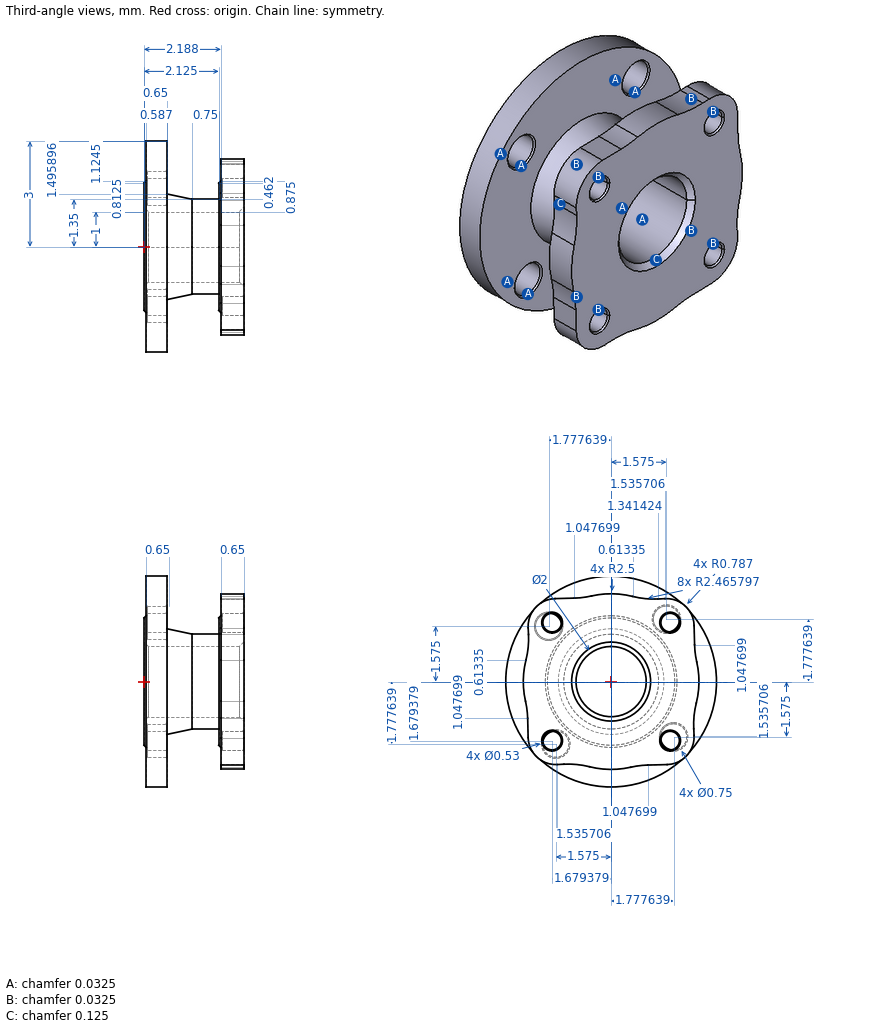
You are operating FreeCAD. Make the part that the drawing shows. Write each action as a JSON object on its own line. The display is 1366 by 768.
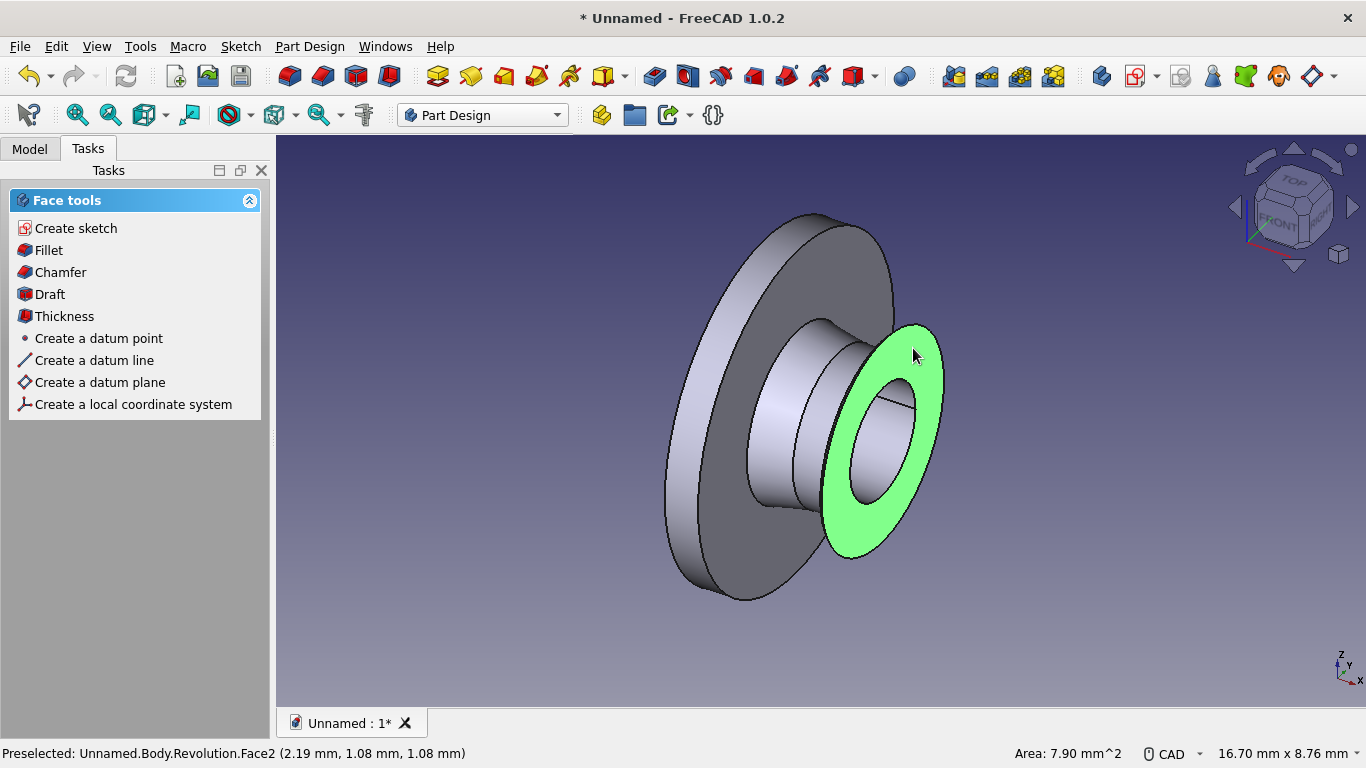
{"action": "left_click", "coordinate": [1134, 76]}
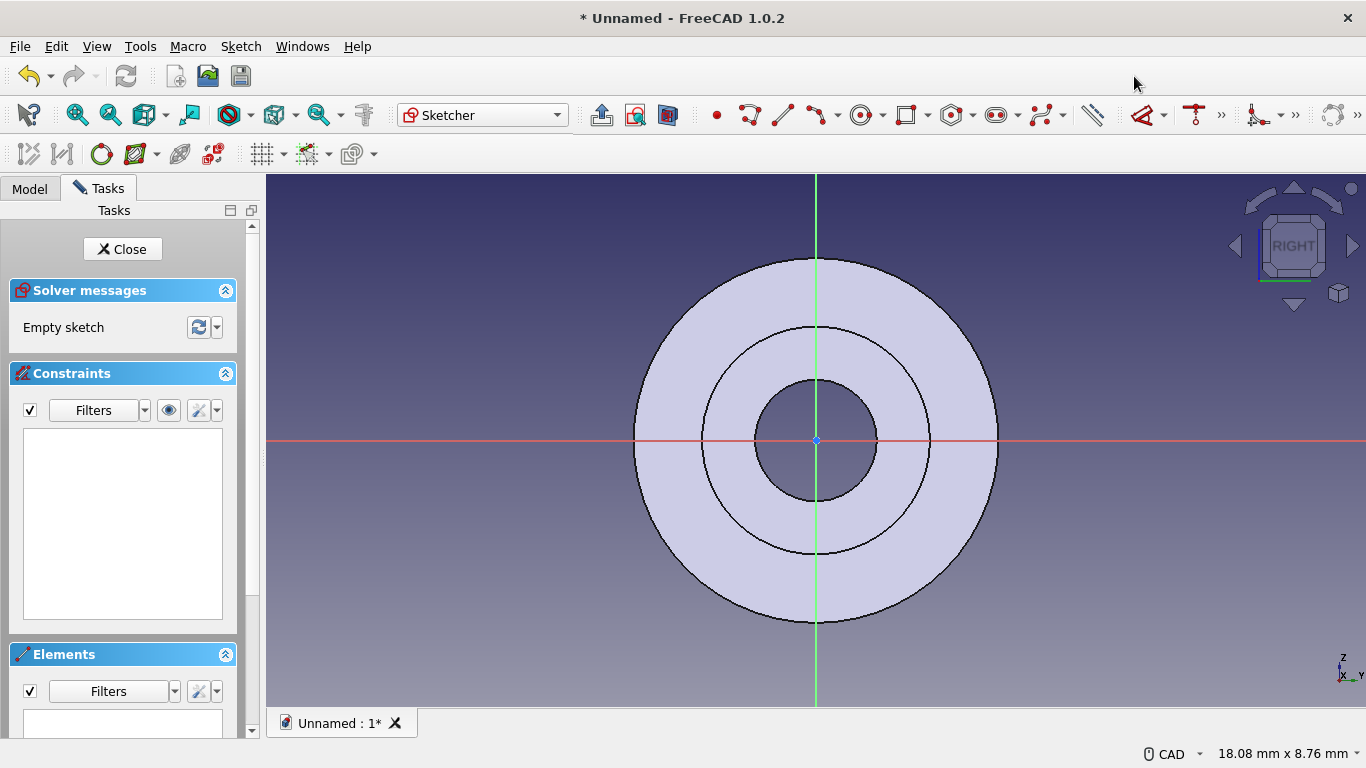
{"action": "left_click", "coordinate": [783, 116]}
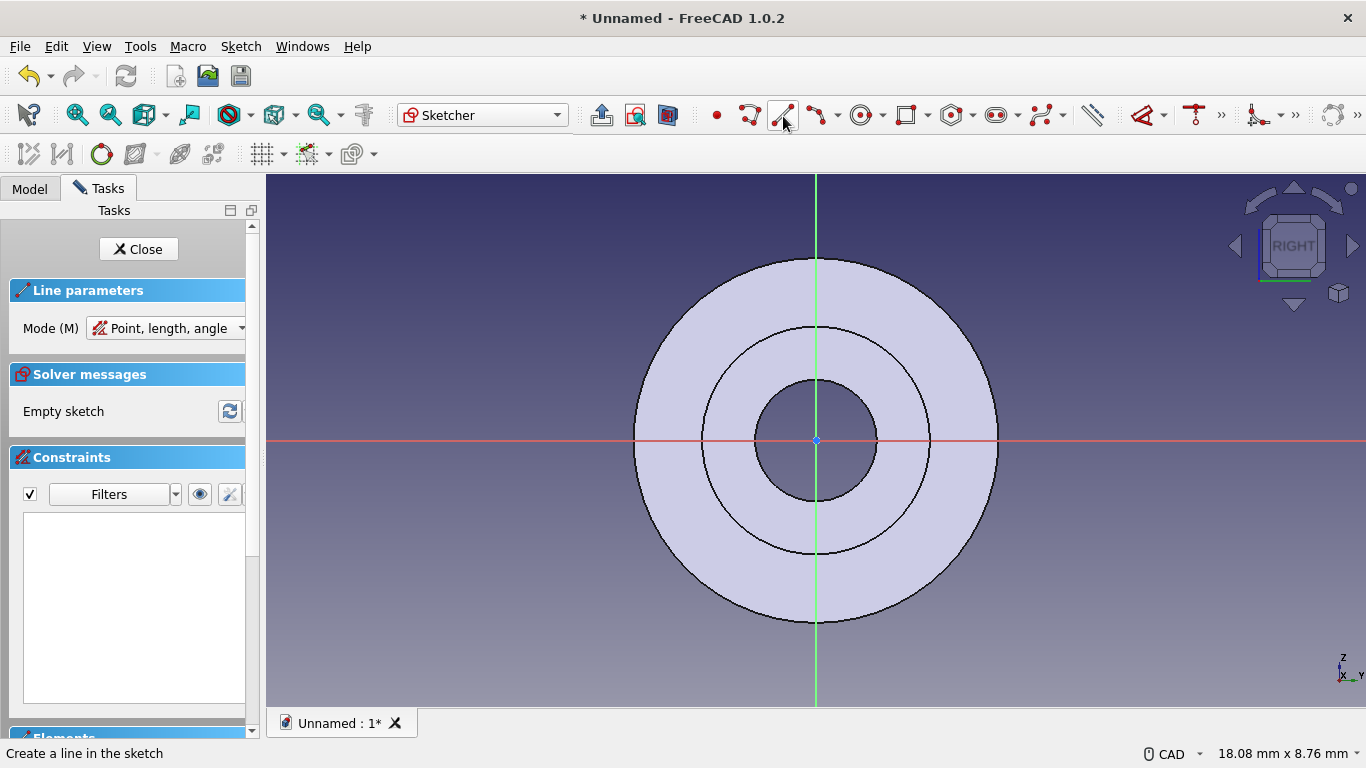
{"action": "left_click", "coordinate": [960, 377]}
{"action": "left_click", "coordinate": [957, 344]}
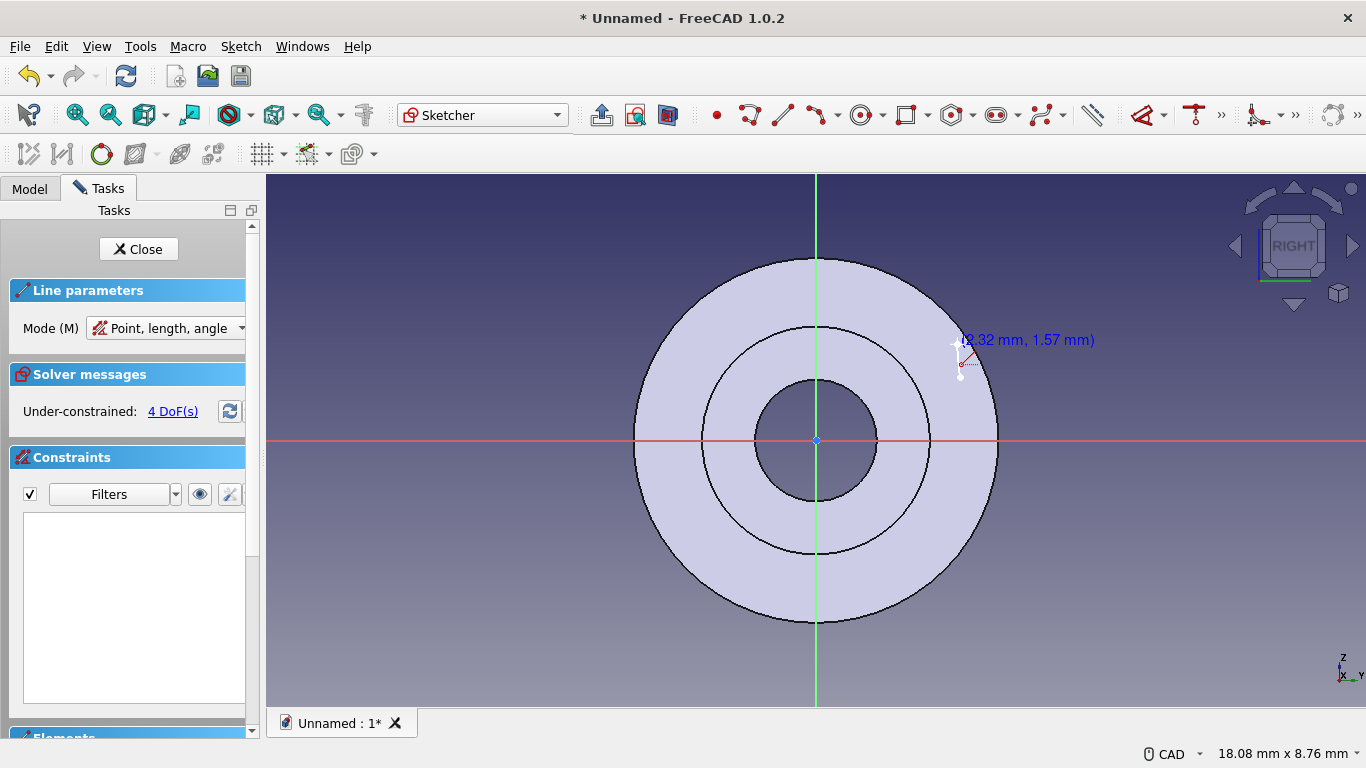
{"action": "left_click", "coordinate": [909, 297]}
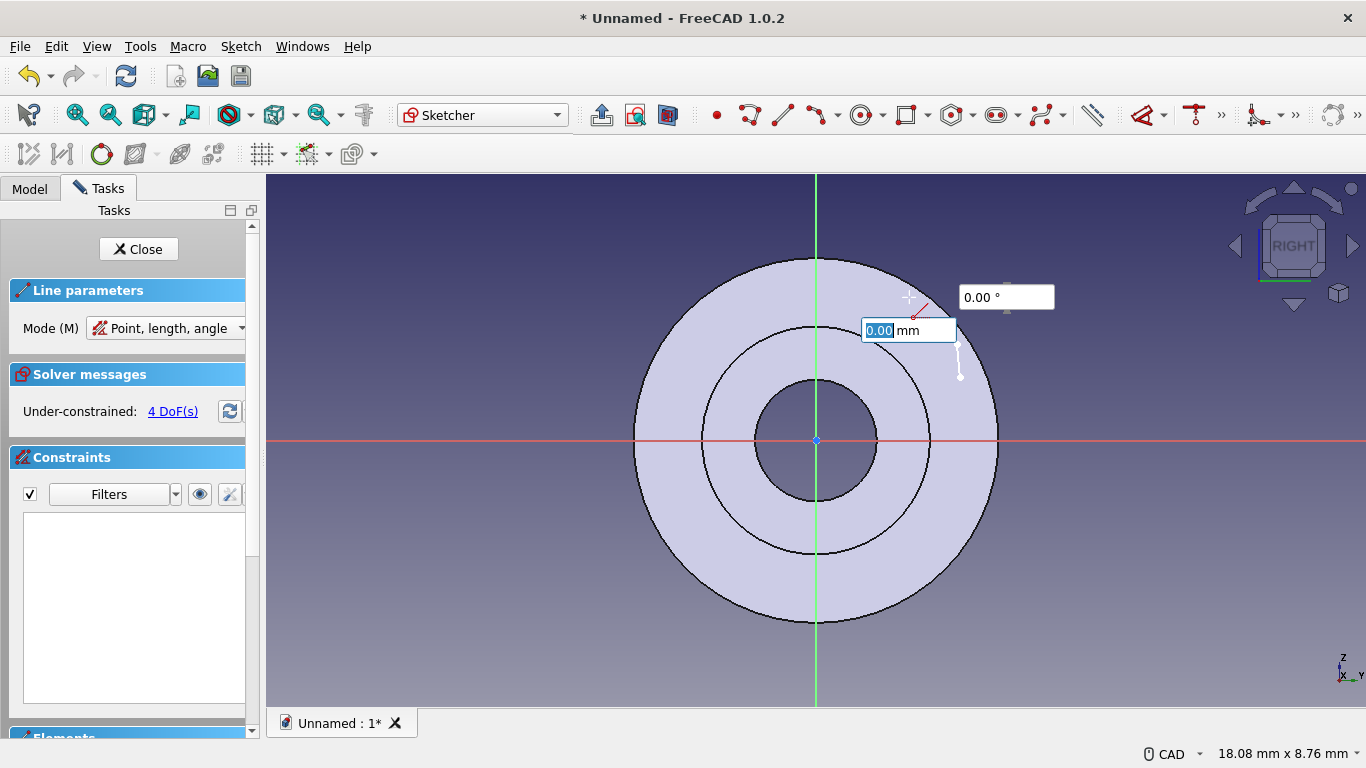
{"action": "scroll", "coordinate": [898, 297], "scroll_direction": "up", "scroll_amount": 2}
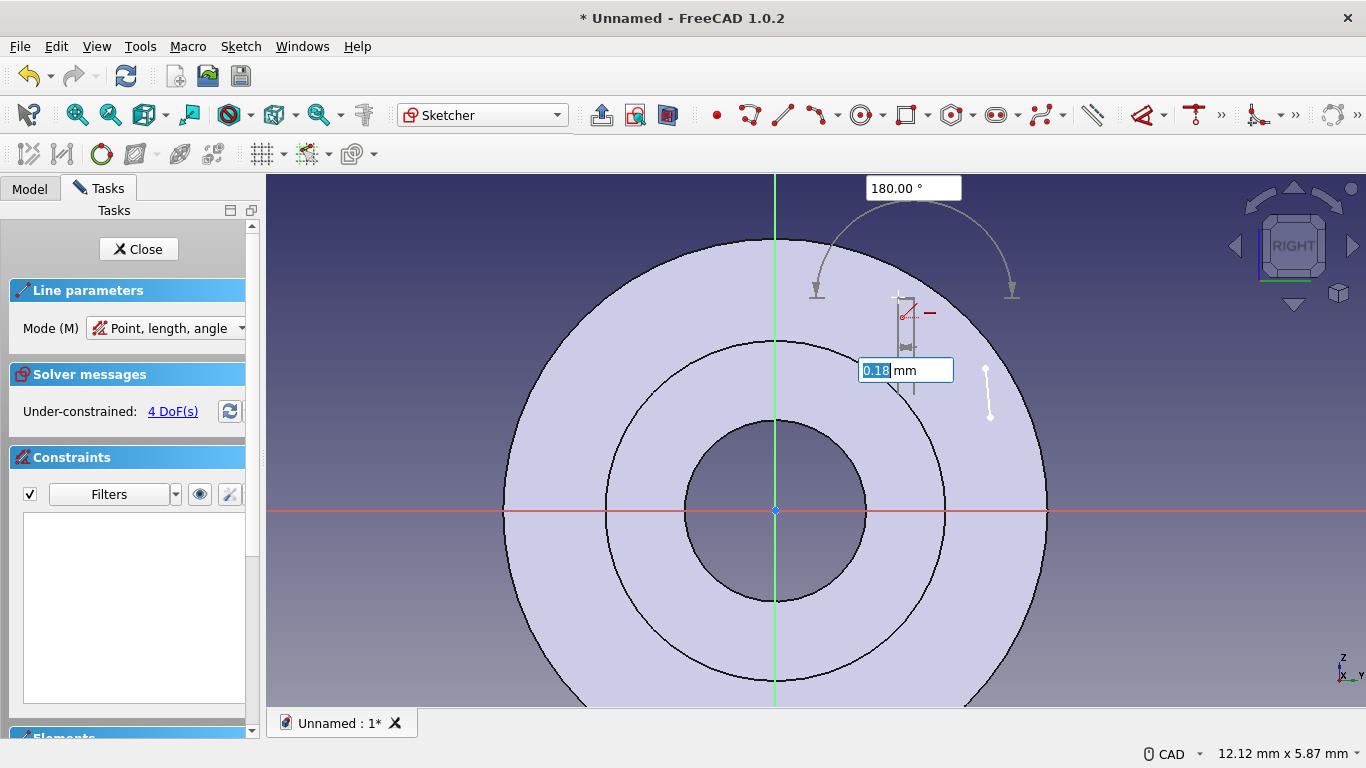
{"action": "left_click", "coordinate": [897, 299]}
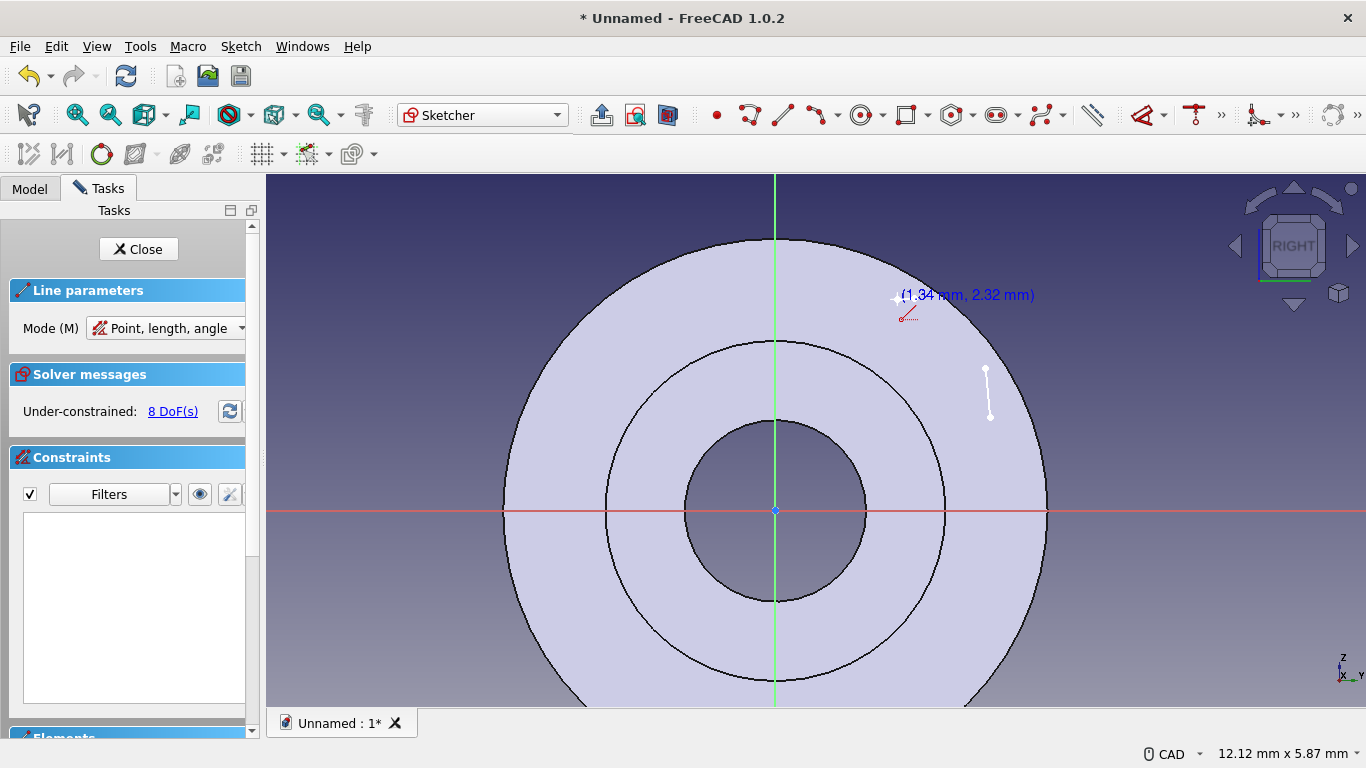
{"action": "left_click", "coordinate": [680, 295]}
{"action": "left_click", "coordinate": [631, 299]}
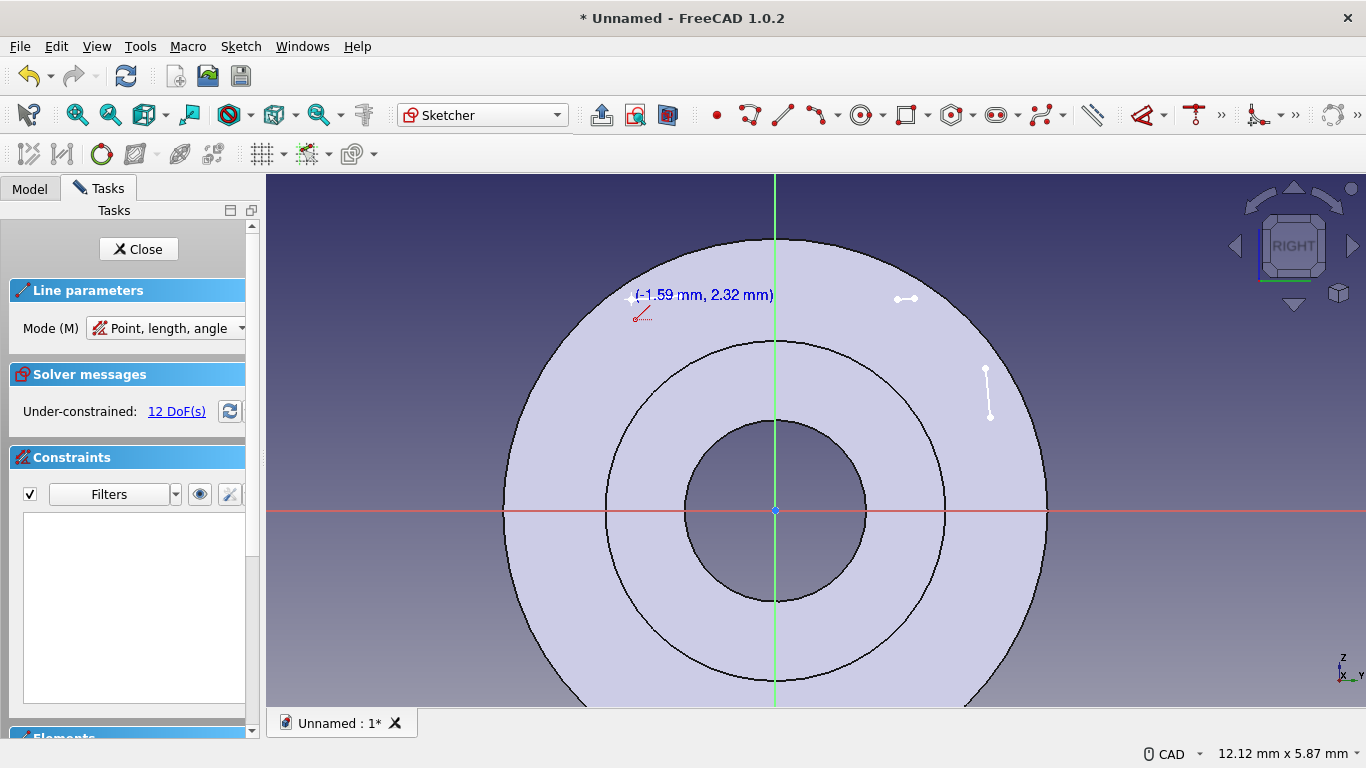
{"action": "left_click", "coordinate": [561, 372]}
{"action": "left_click", "coordinate": [563, 389]}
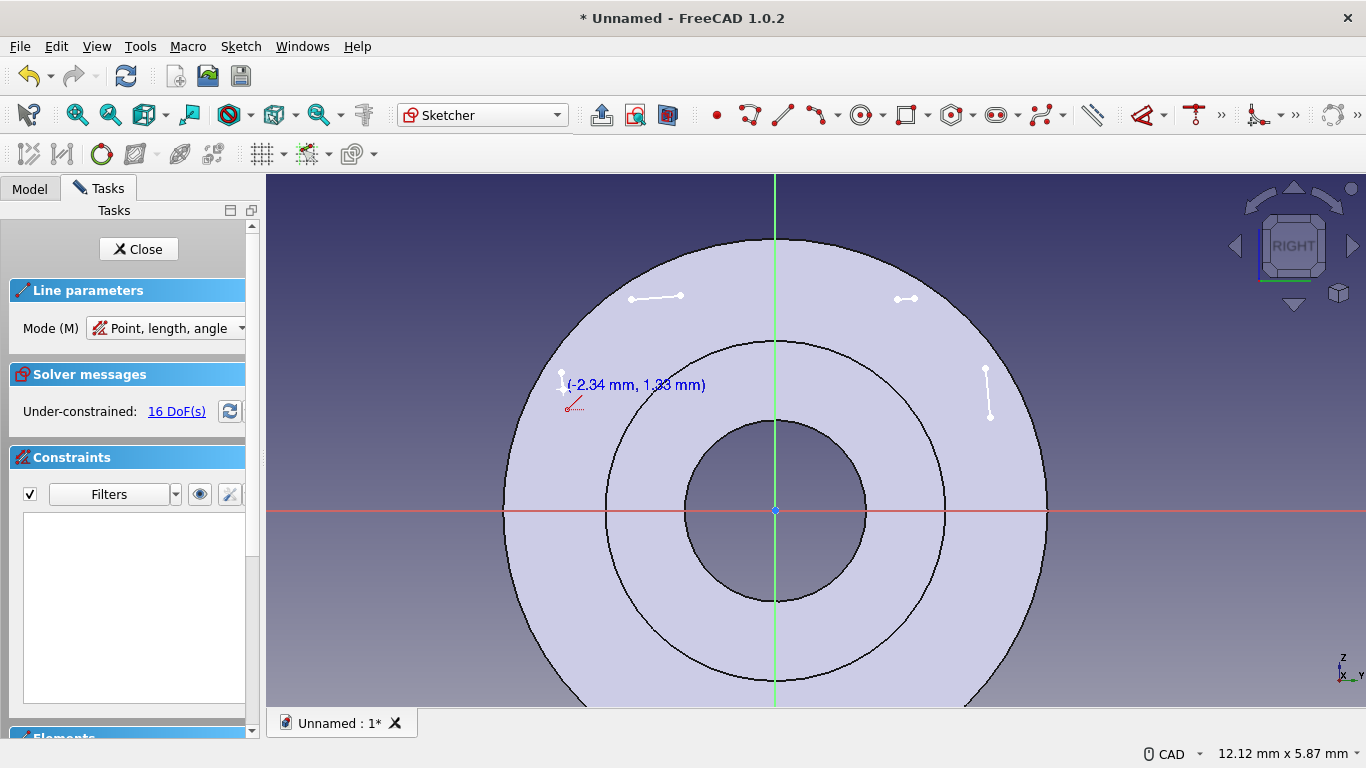
{"action": "left_click", "coordinate": [560, 606]}
{"action": "left_click", "coordinate": [564, 656]}